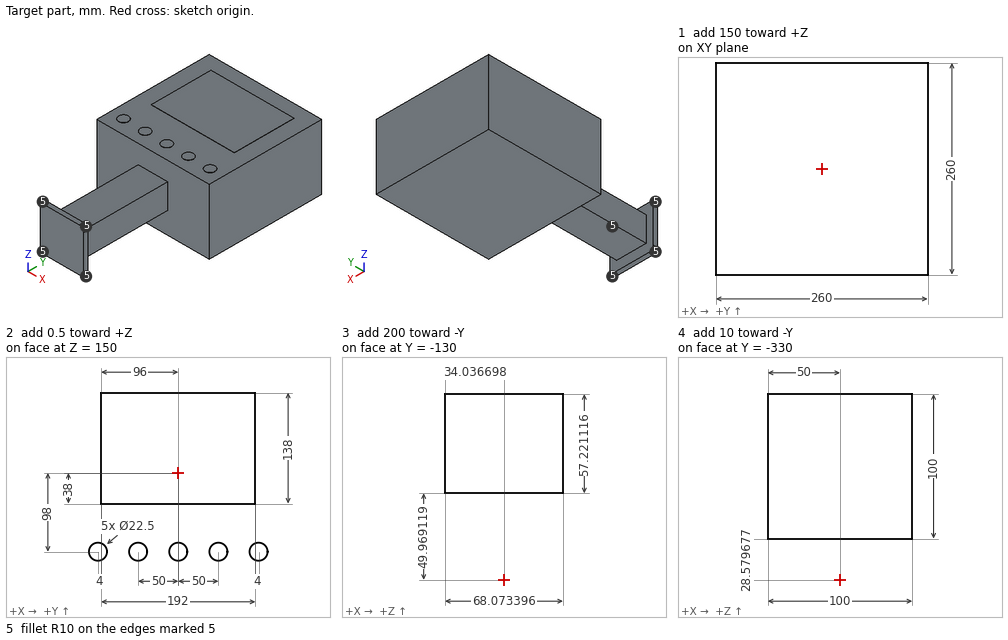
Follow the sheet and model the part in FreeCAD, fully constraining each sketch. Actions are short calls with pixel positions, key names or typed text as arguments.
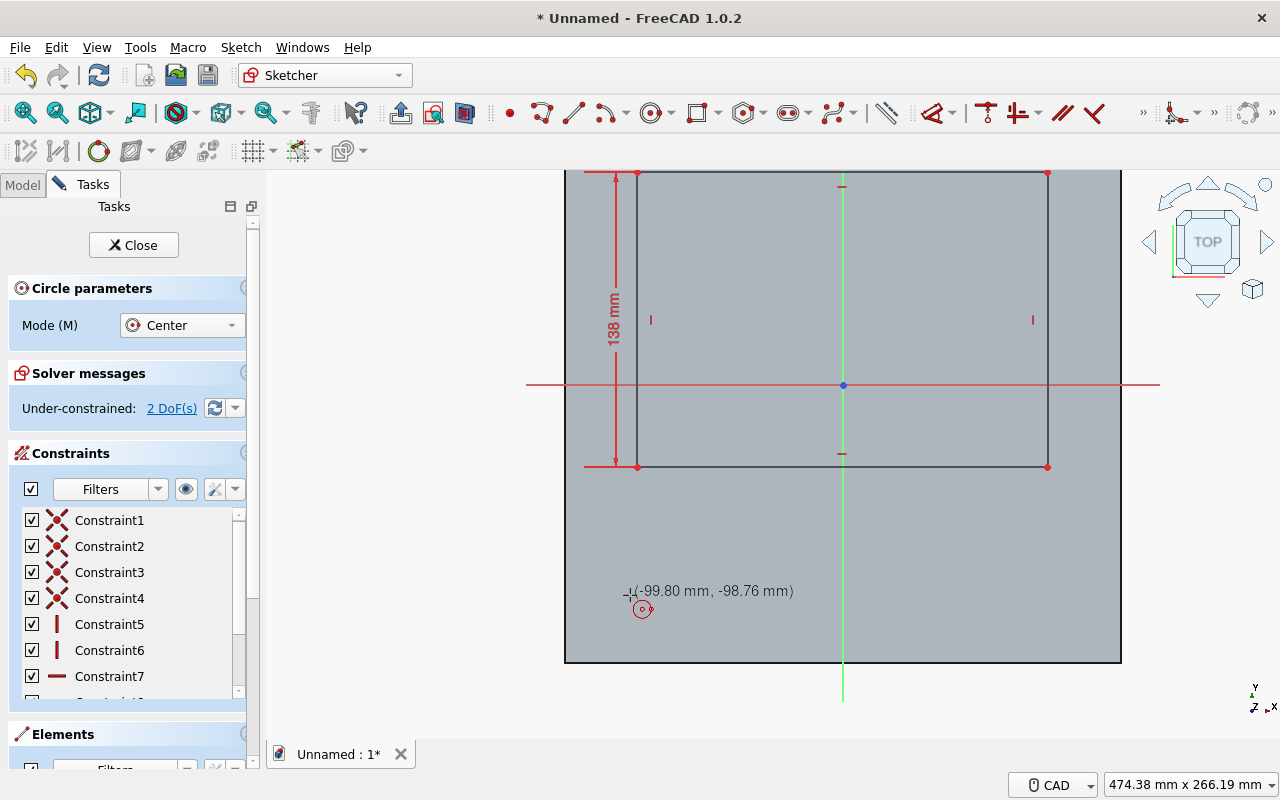
click(629, 595)
move(646, 578)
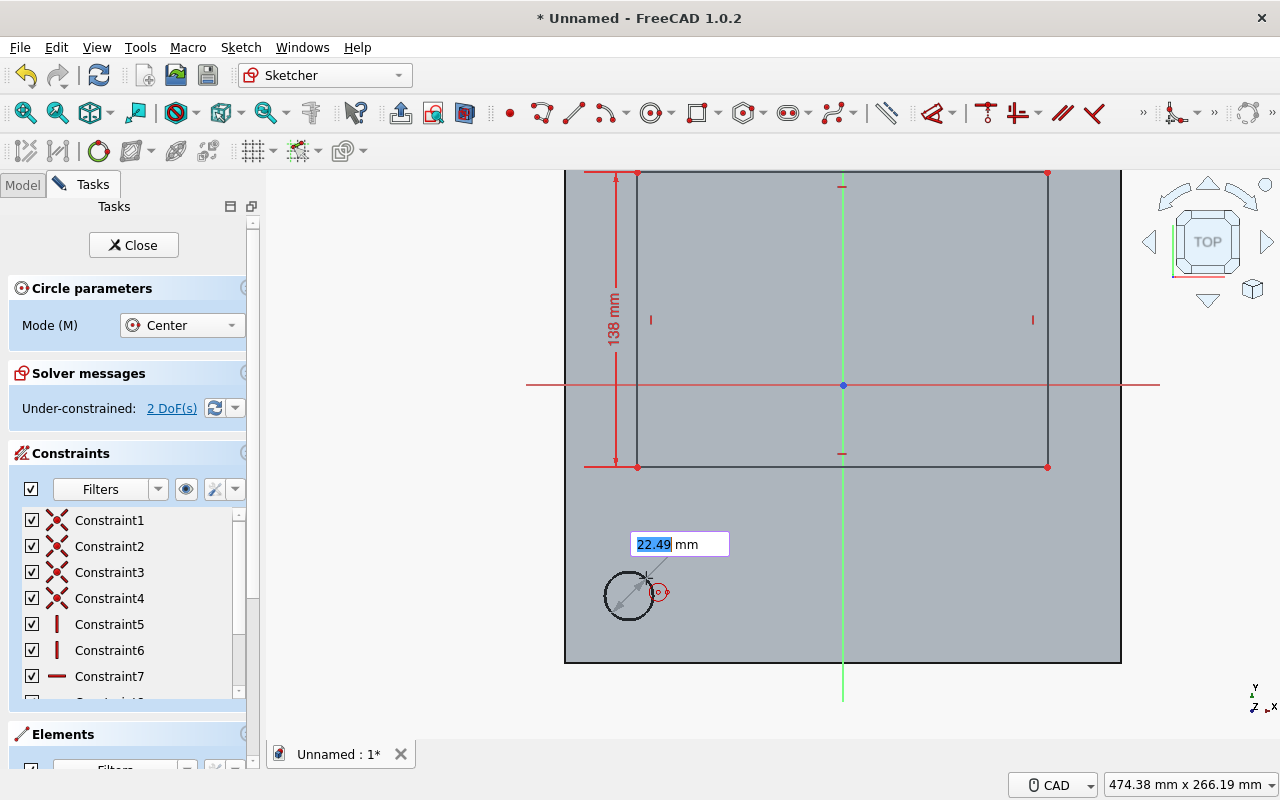
text(22.5)
key(Return)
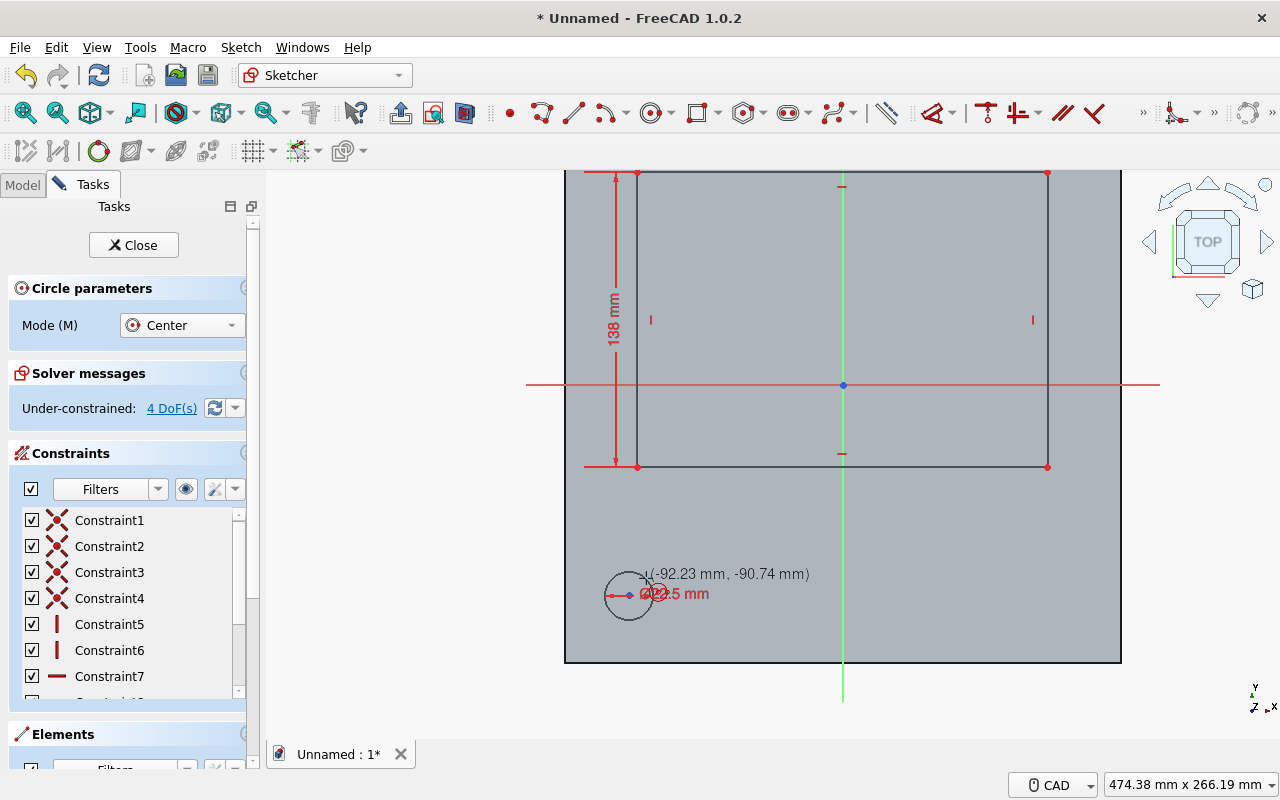
click(736, 595)
move(753, 578)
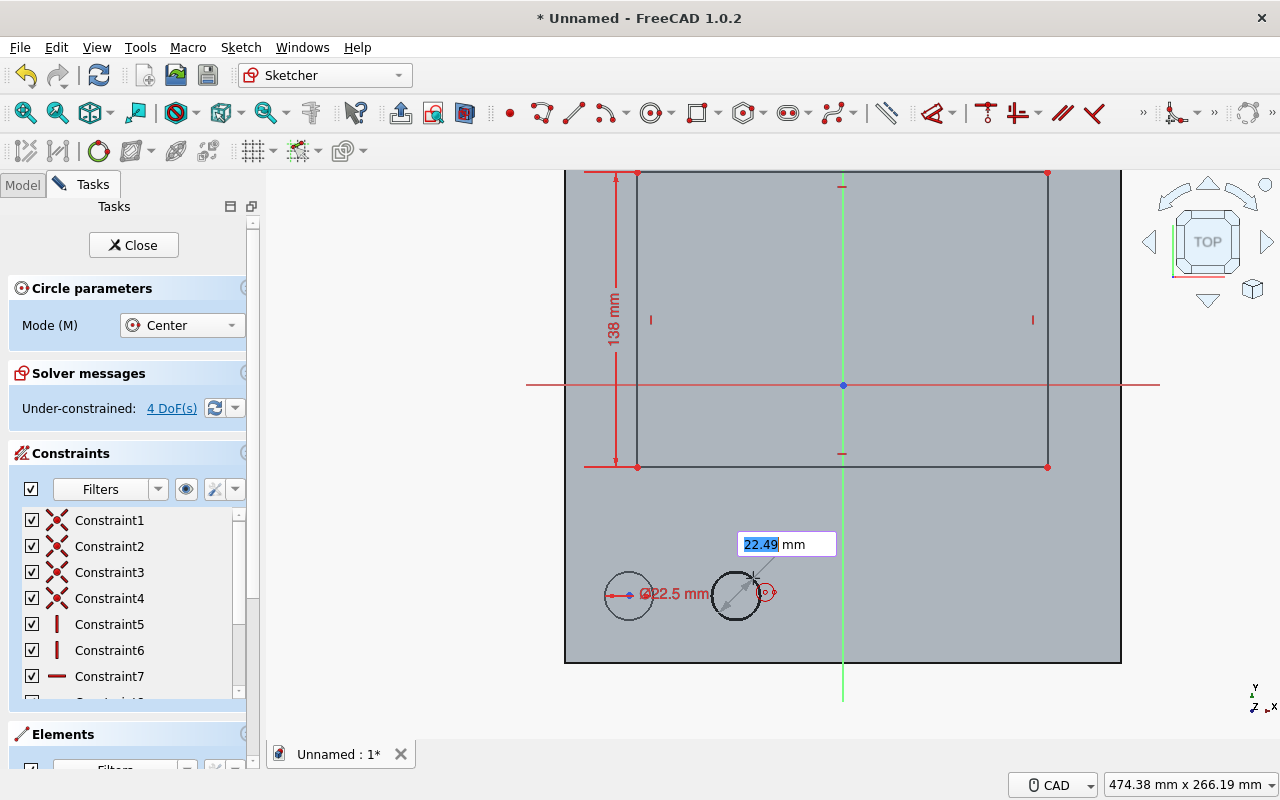
text(22.5)
key(Return)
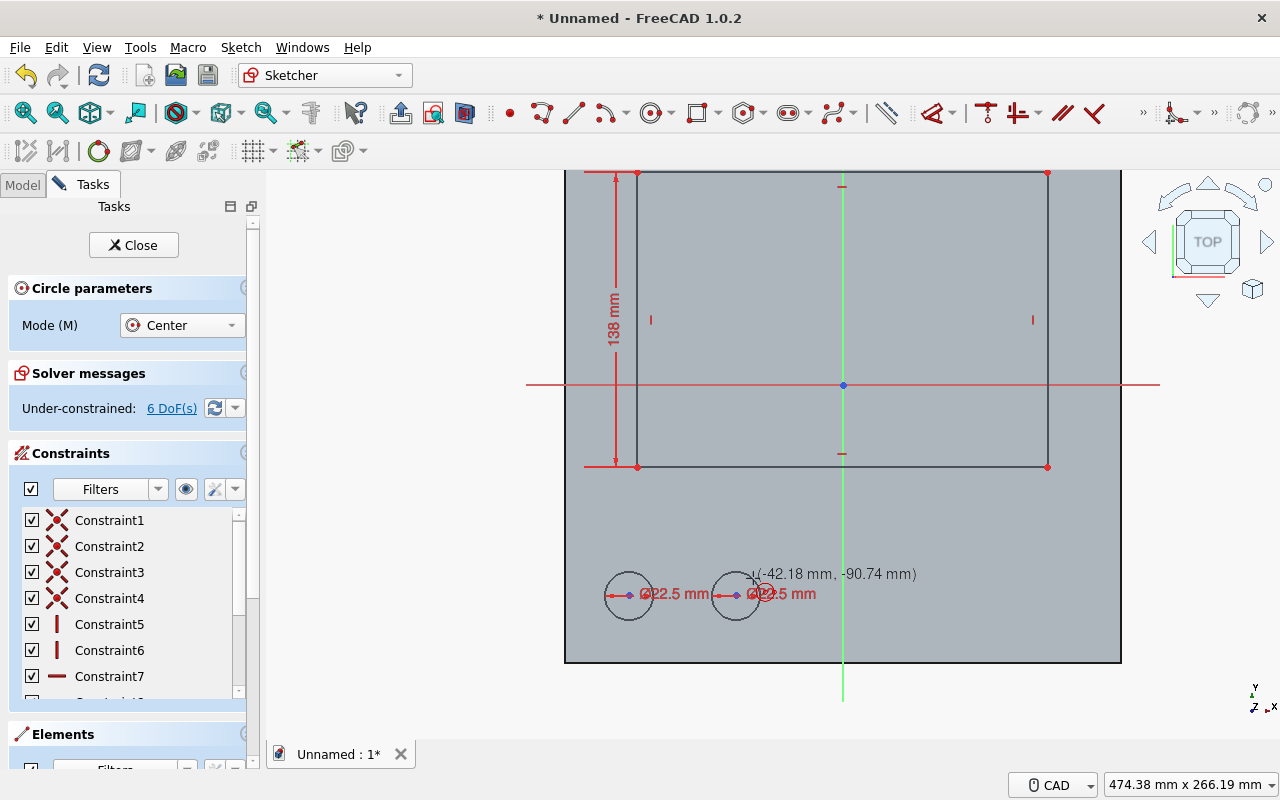
click(950, 595)
move(967, 578)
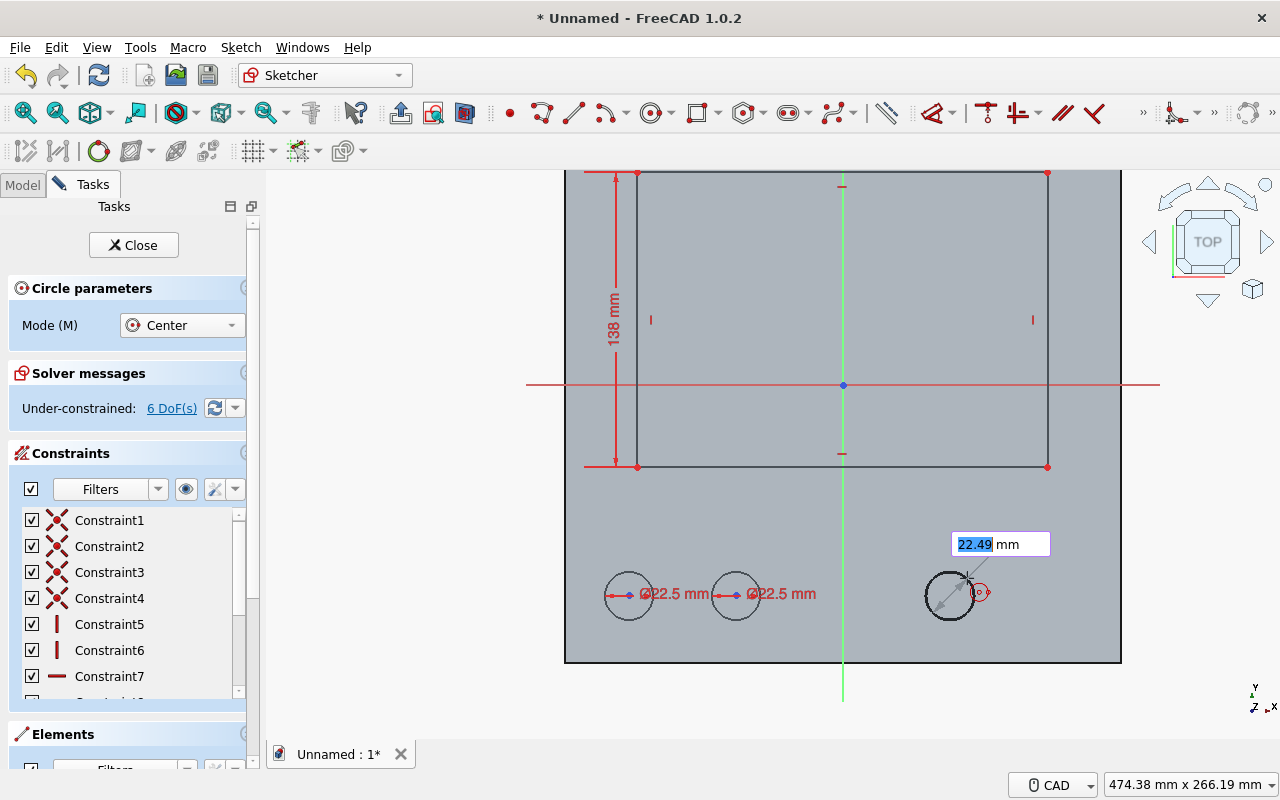
text(22.5)
key(Return)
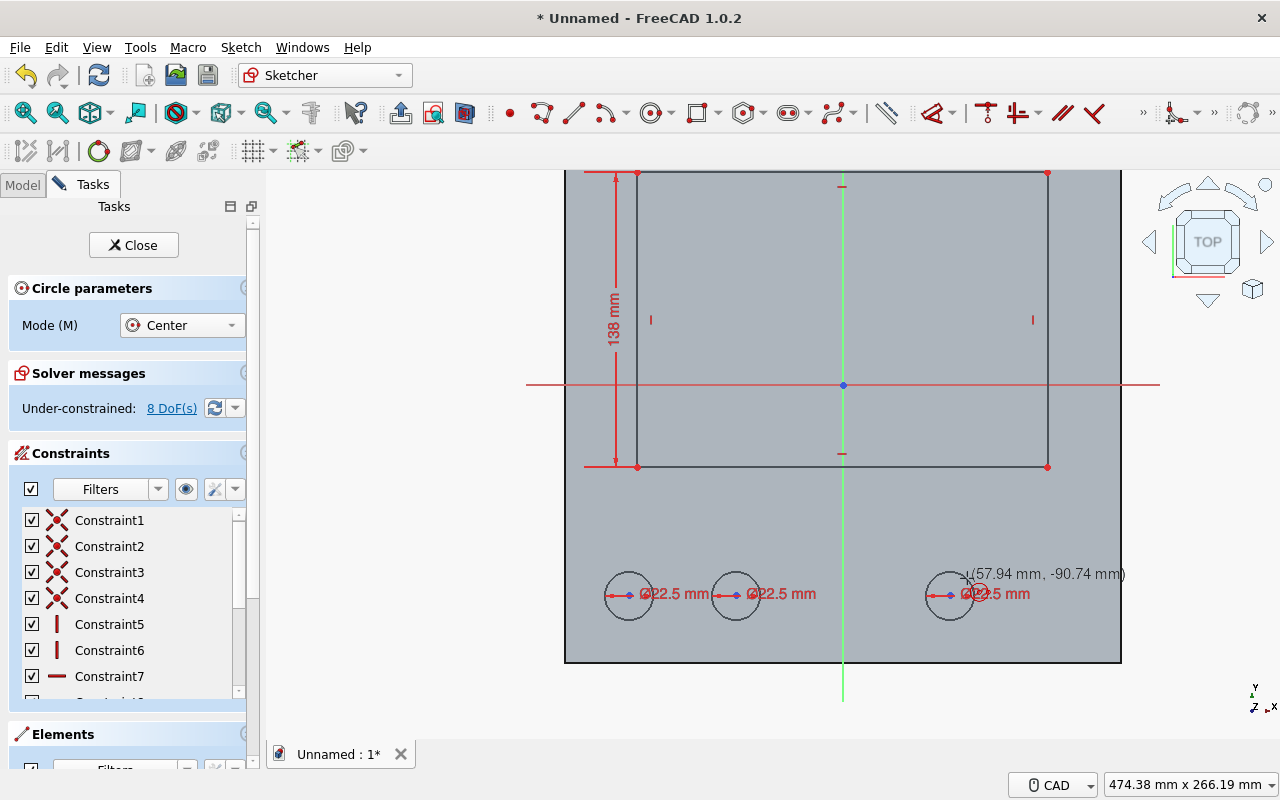
click(1057, 595)
move(1074, 578)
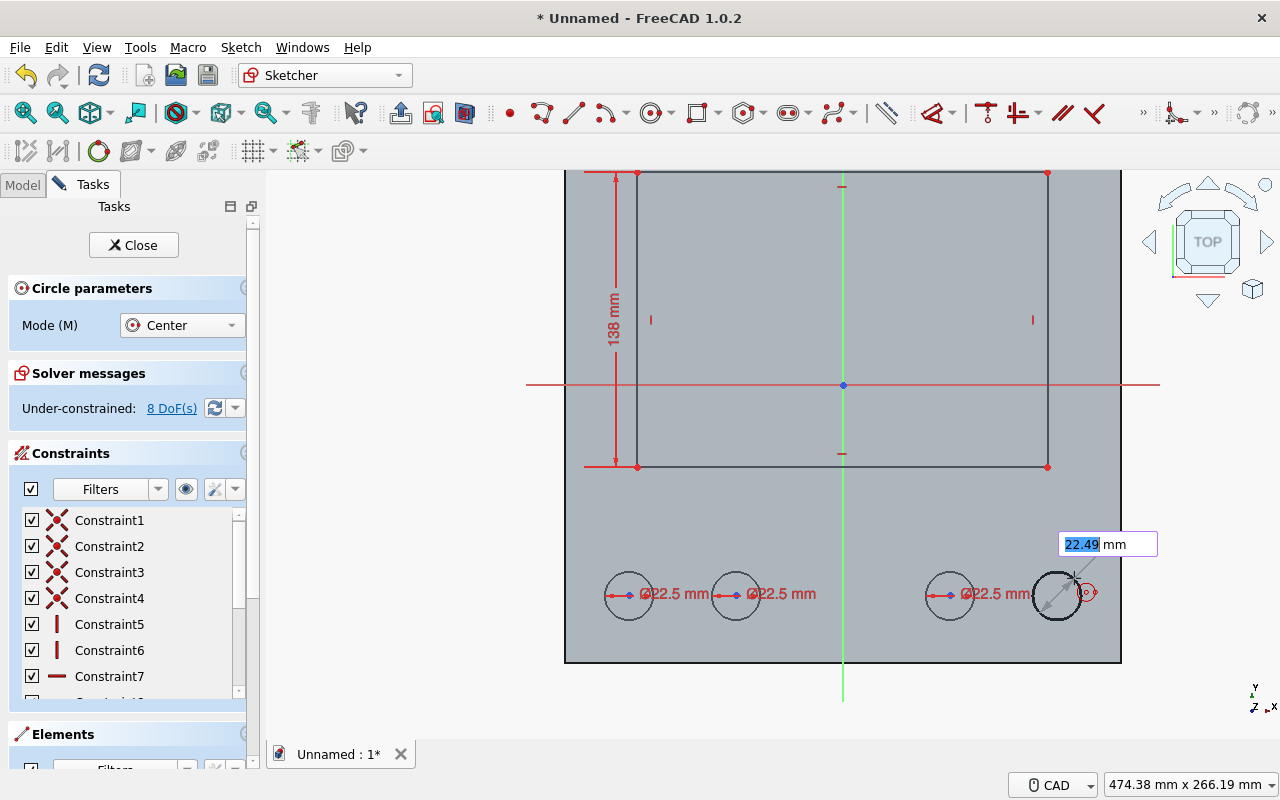
text(22.5)
key(Return)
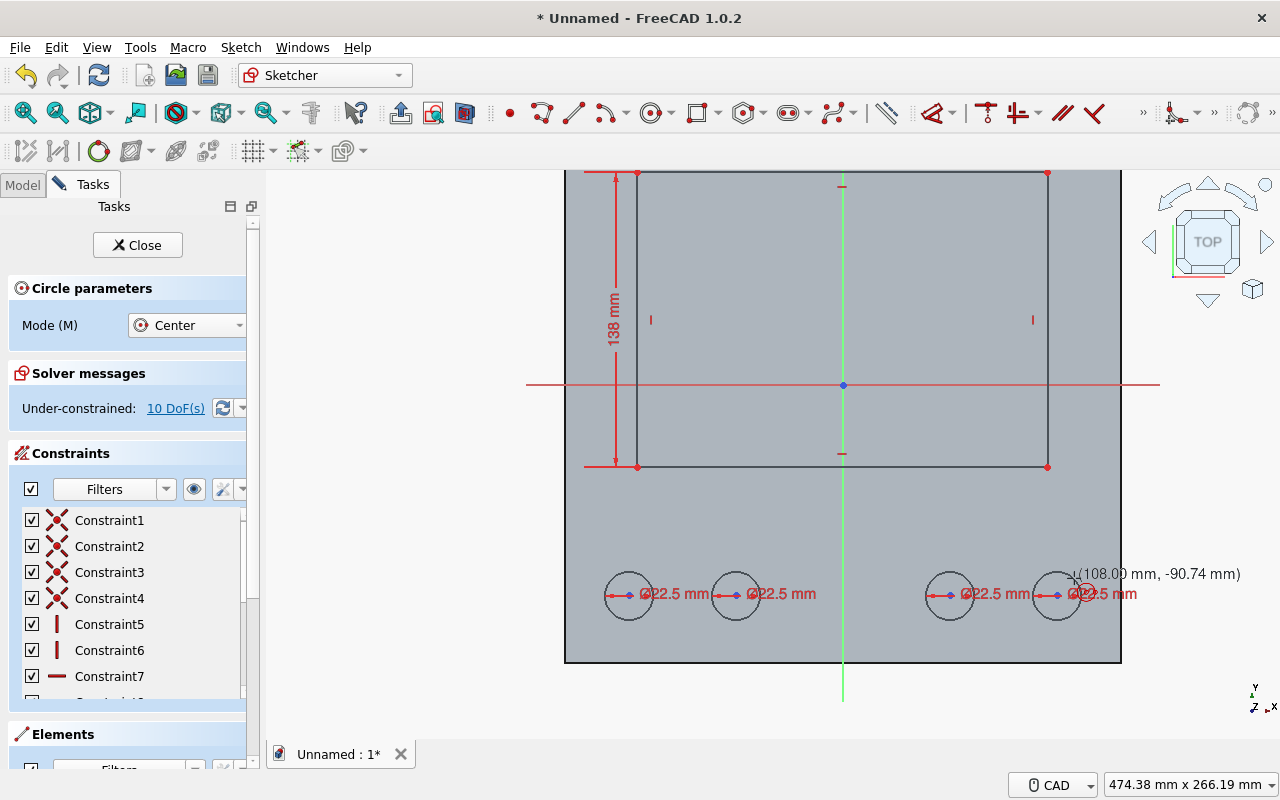
click(843, 595)
move(860, 578)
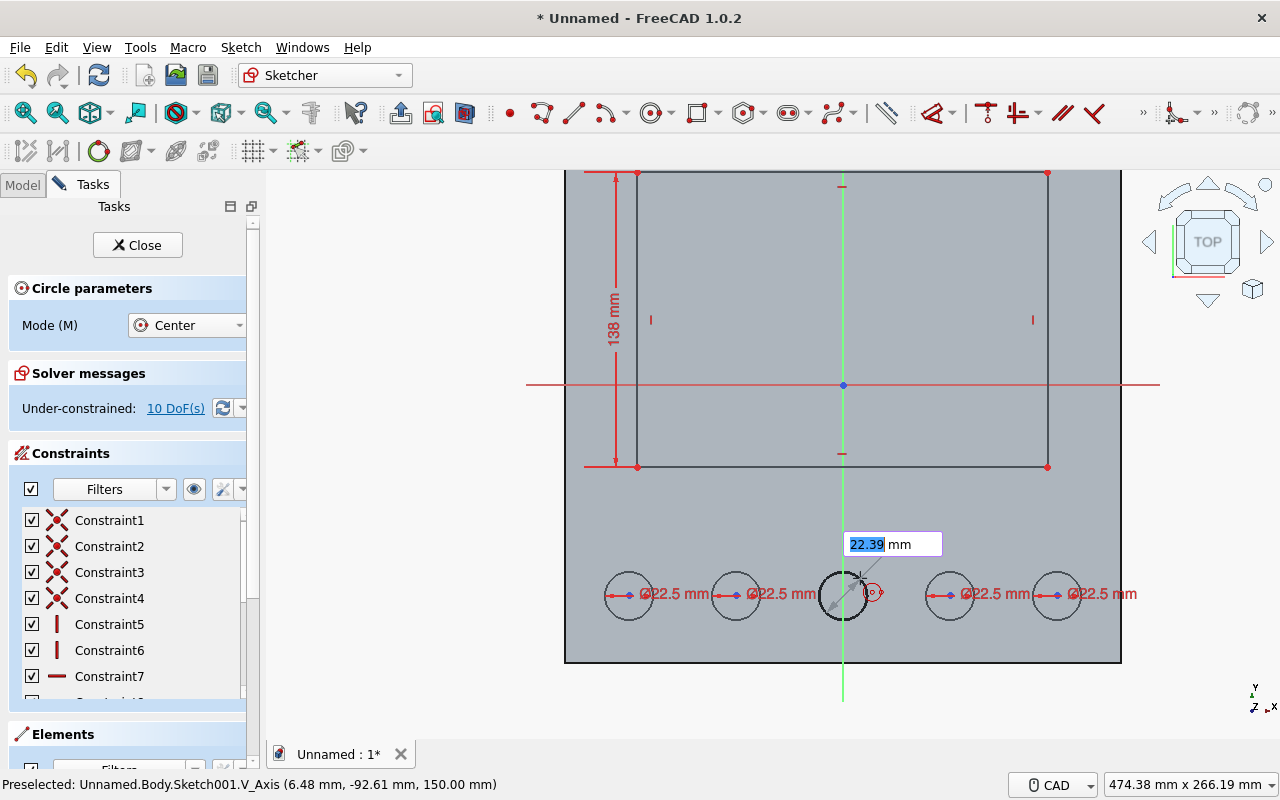
text(22.5)
key(Return)
key(Escape)